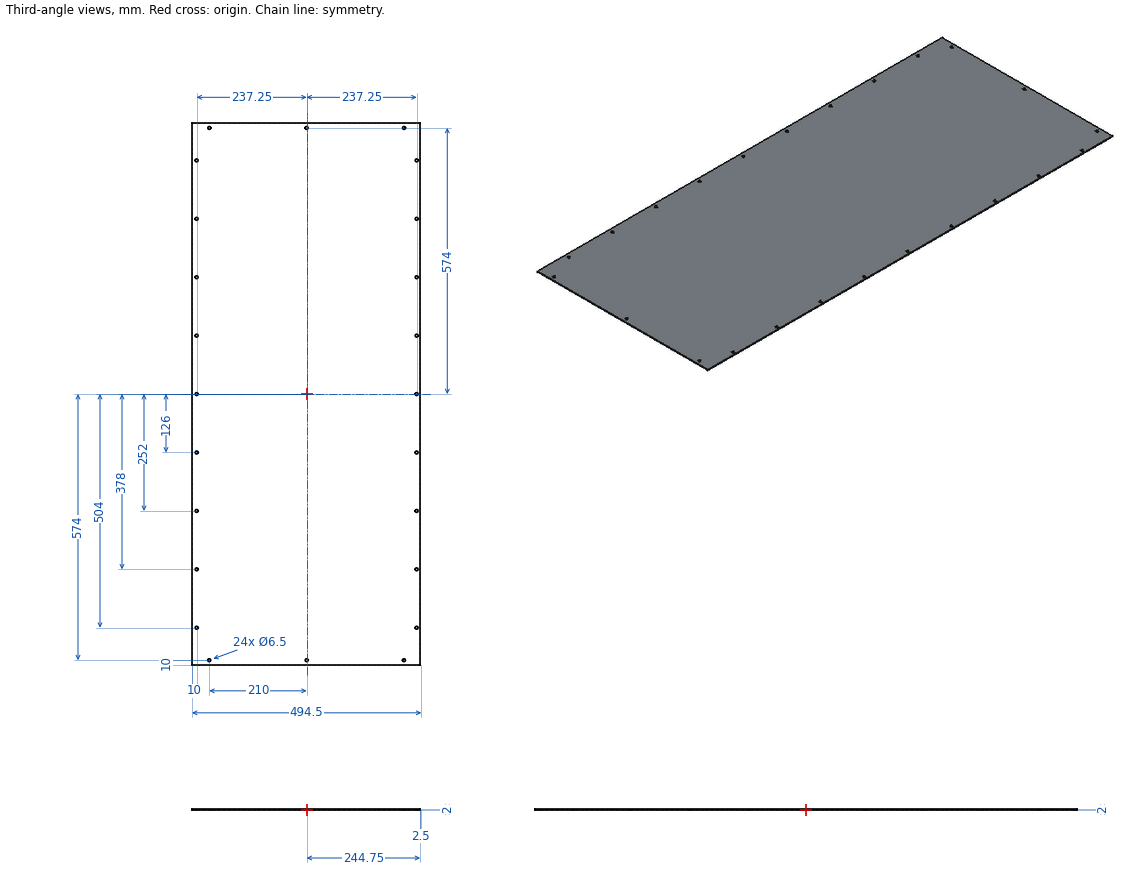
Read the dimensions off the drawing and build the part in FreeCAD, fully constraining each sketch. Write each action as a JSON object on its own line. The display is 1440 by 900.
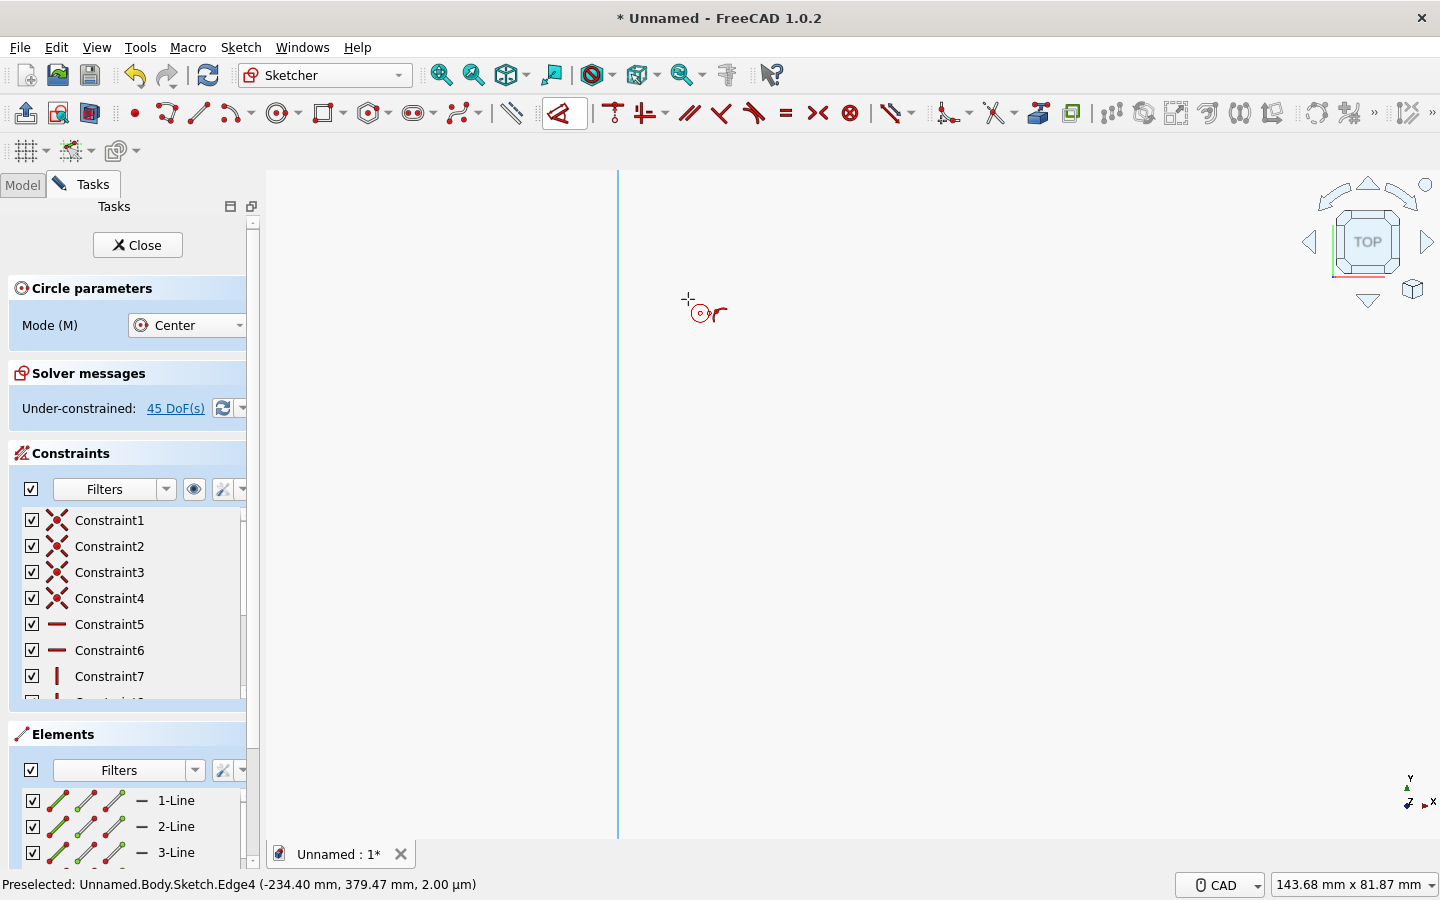
{"action": "scroll", "coordinate": [688, 299], "scroll_direction": "down", "scroll_amount": 15}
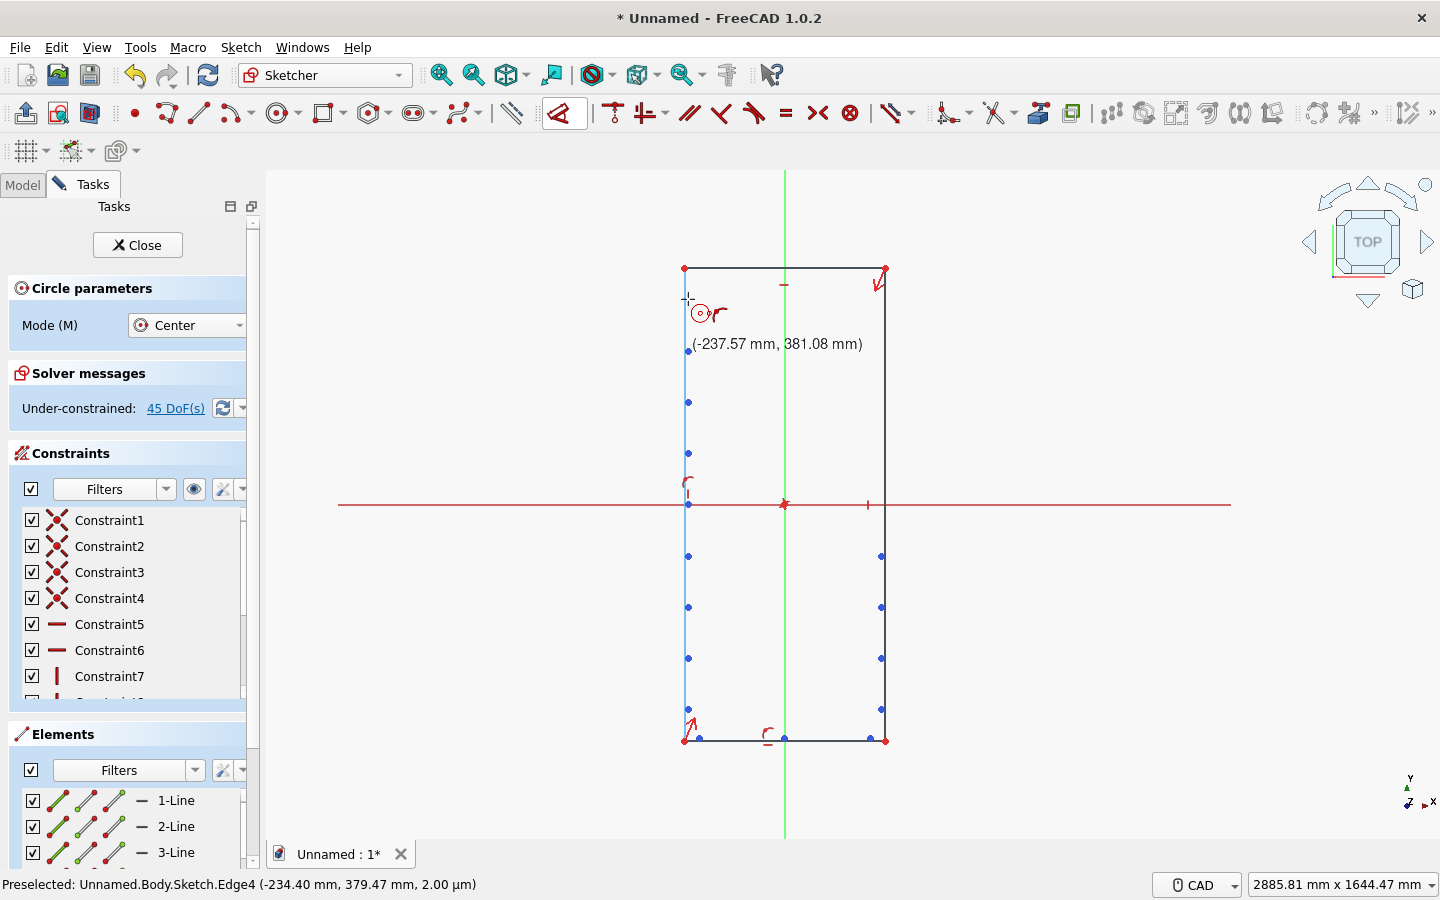
{"action": "scroll", "coordinate": [688, 299], "scroll_direction": "up", "scroll_amount": 7}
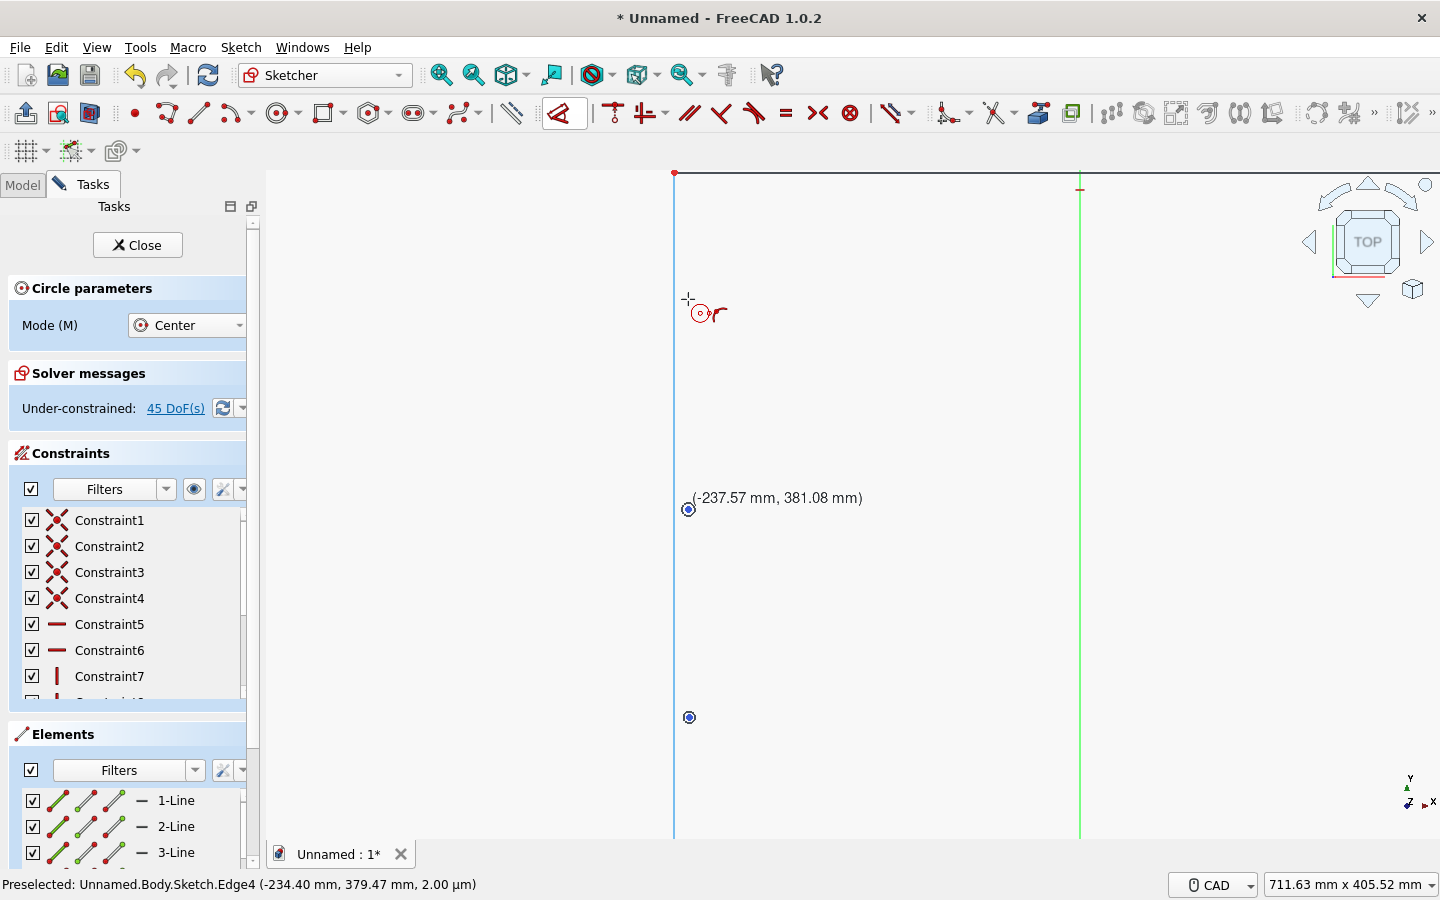
{"action": "left_click", "coordinate": [689, 300]}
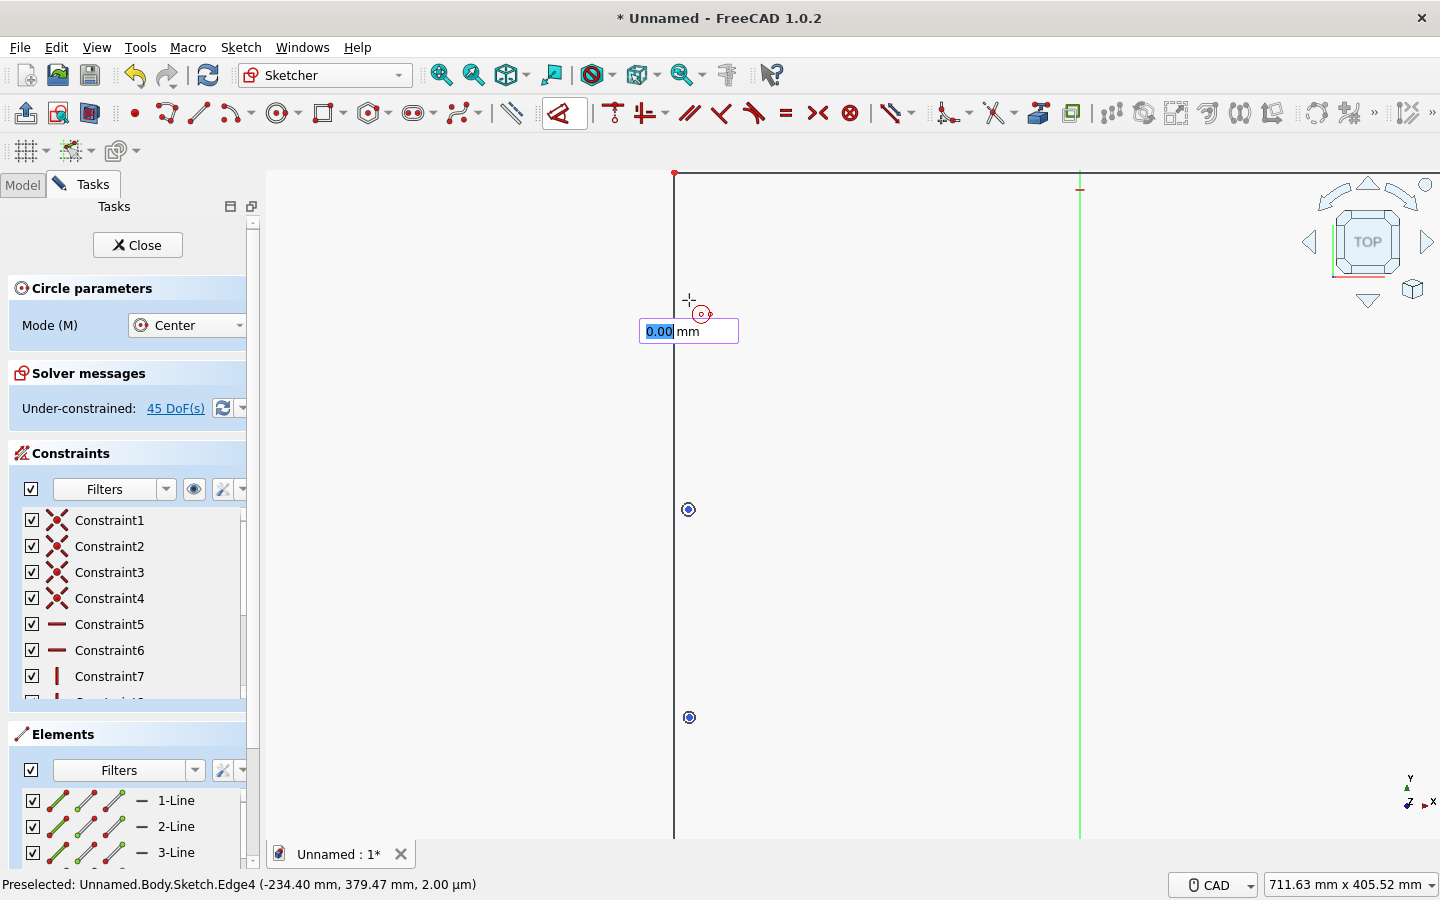
{"action": "scroll", "coordinate": [693, 297], "scroll_direction": "up", "scroll_amount": 6}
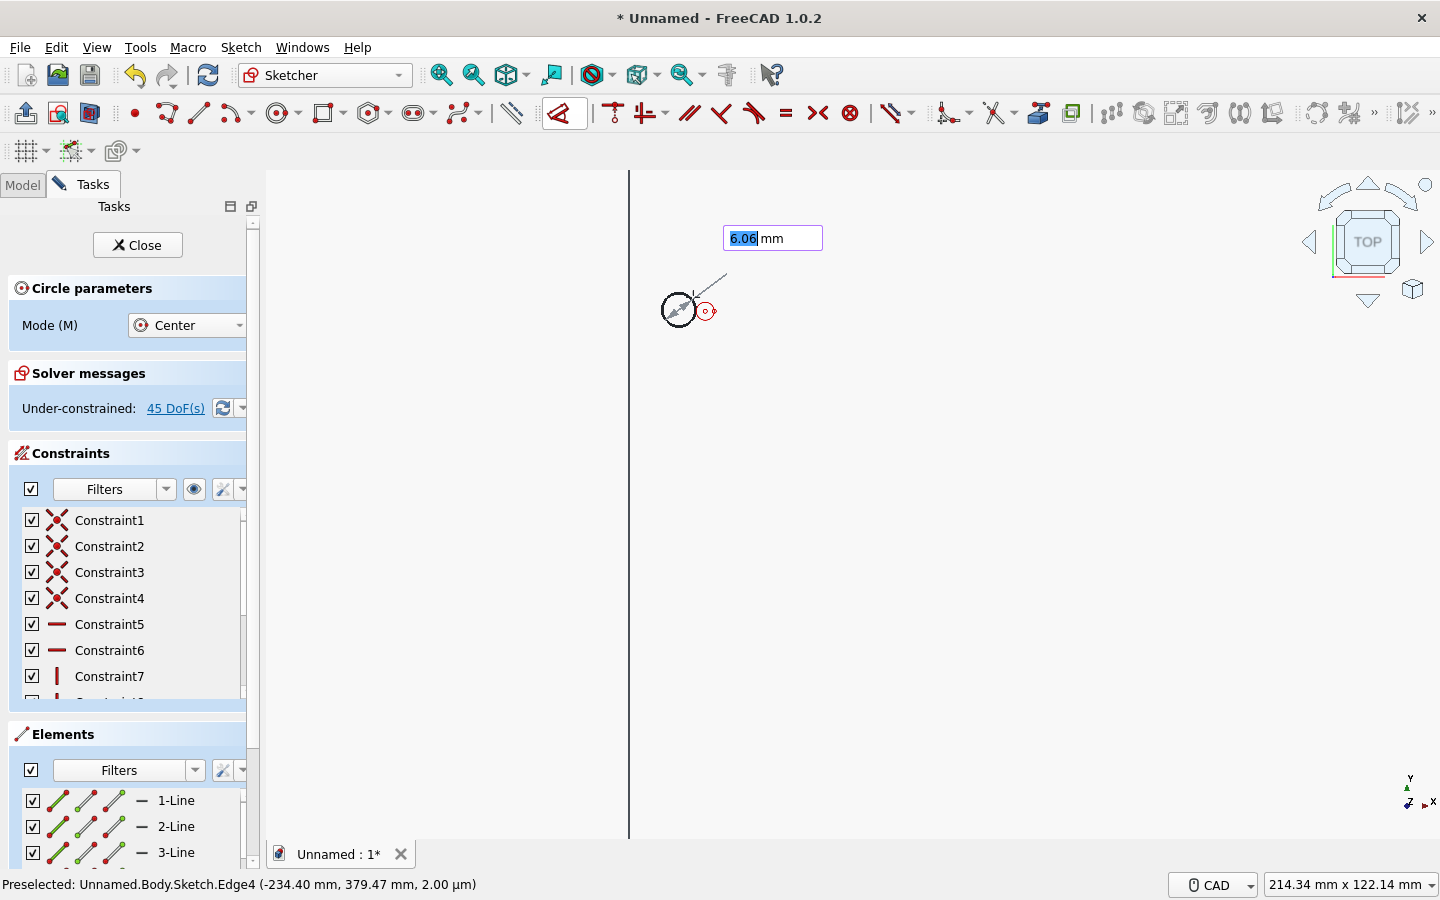
{"action": "left_click", "coordinate": [691, 295]}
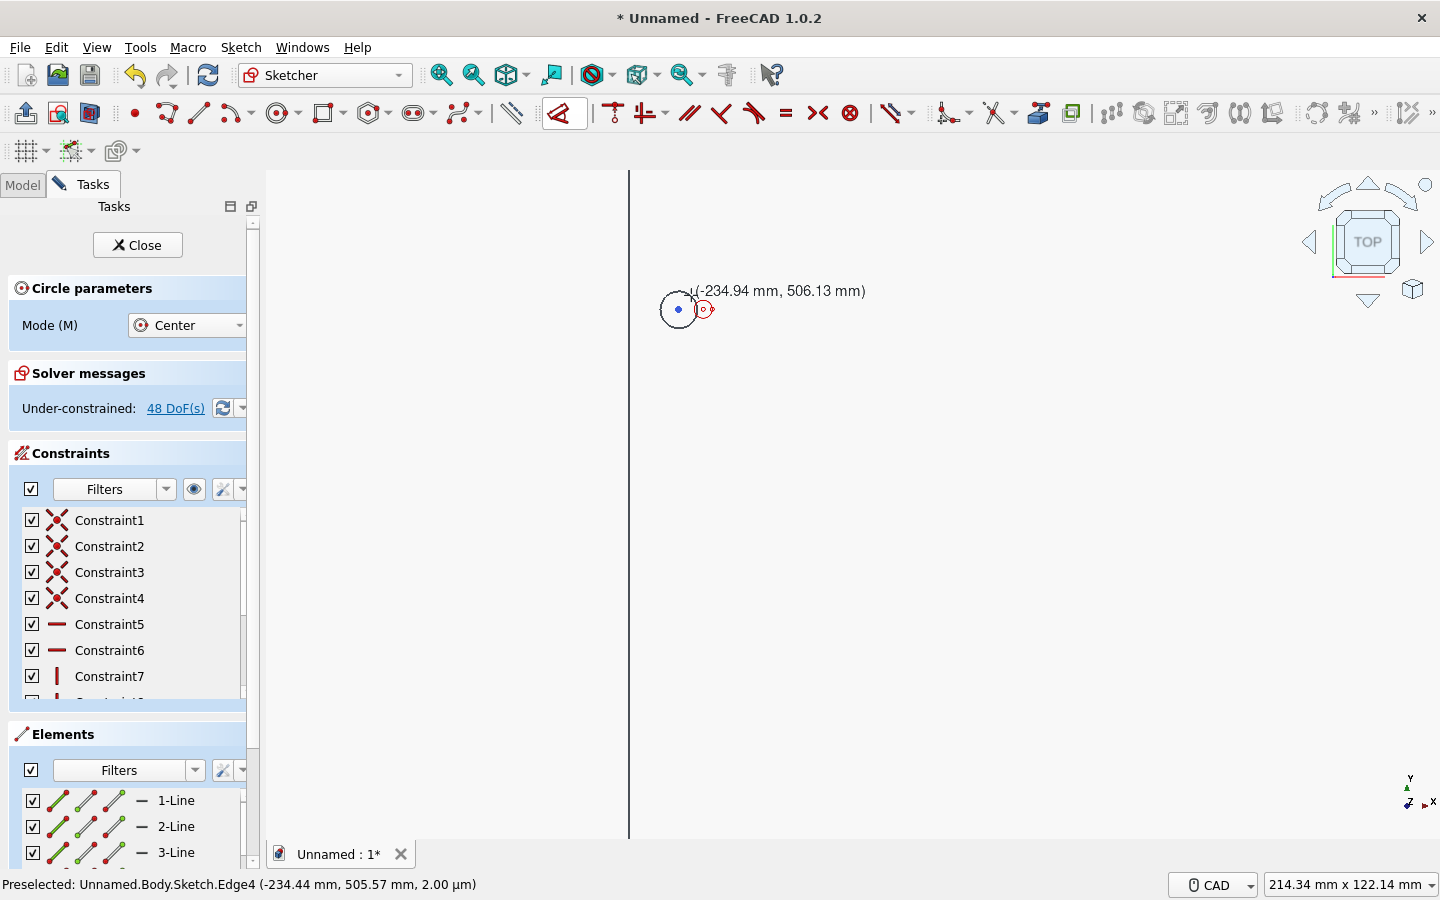
{"action": "scroll", "coordinate": [689, 299], "scroll_direction": "down", "scroll_amount": 13}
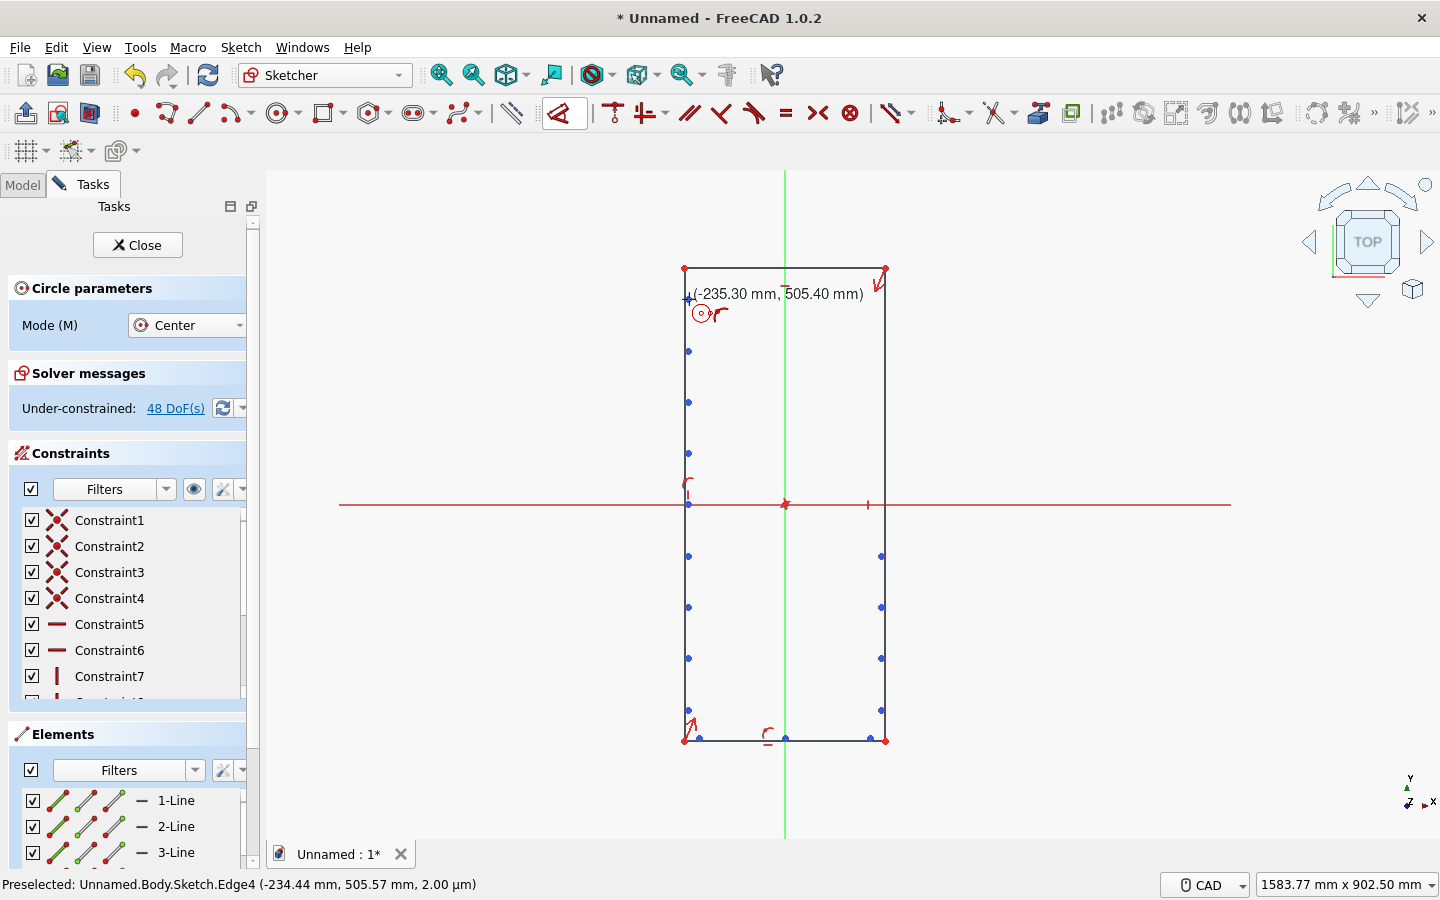
{"action": "scroll", "coordinate": [700, 271], "scroll_direction": "up", "scroll_amount": 15}